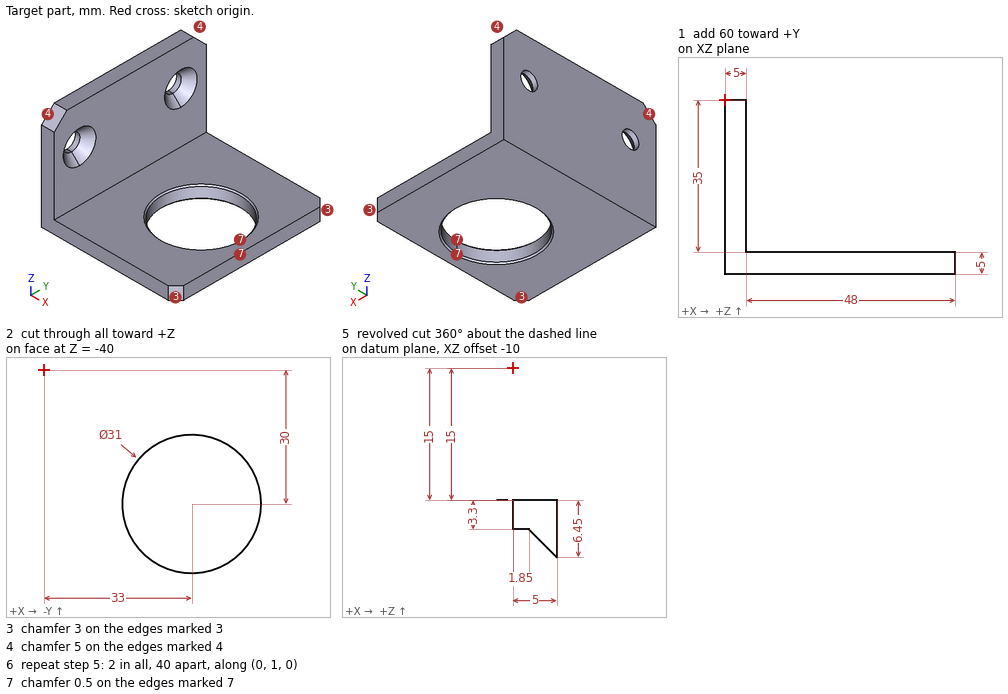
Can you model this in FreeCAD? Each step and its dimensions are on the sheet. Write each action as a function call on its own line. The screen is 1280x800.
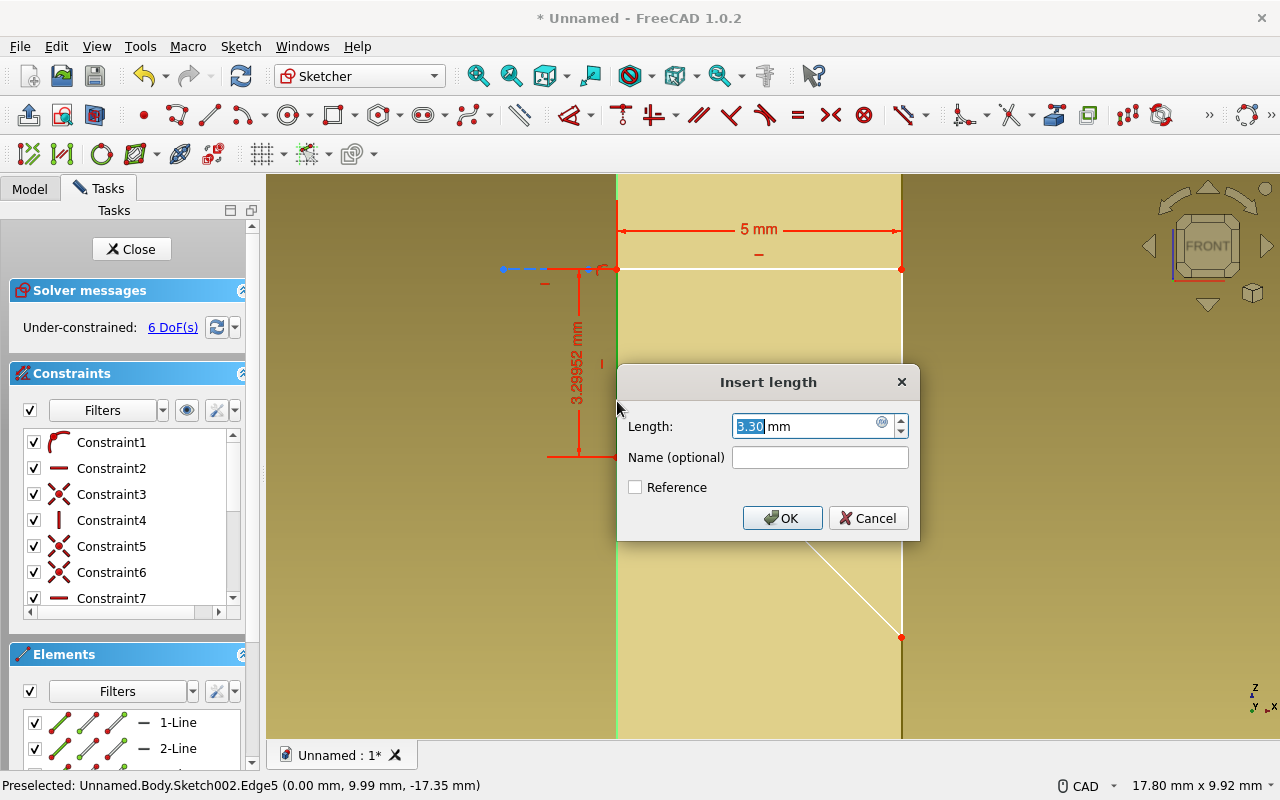
text(3.3)
key(Return)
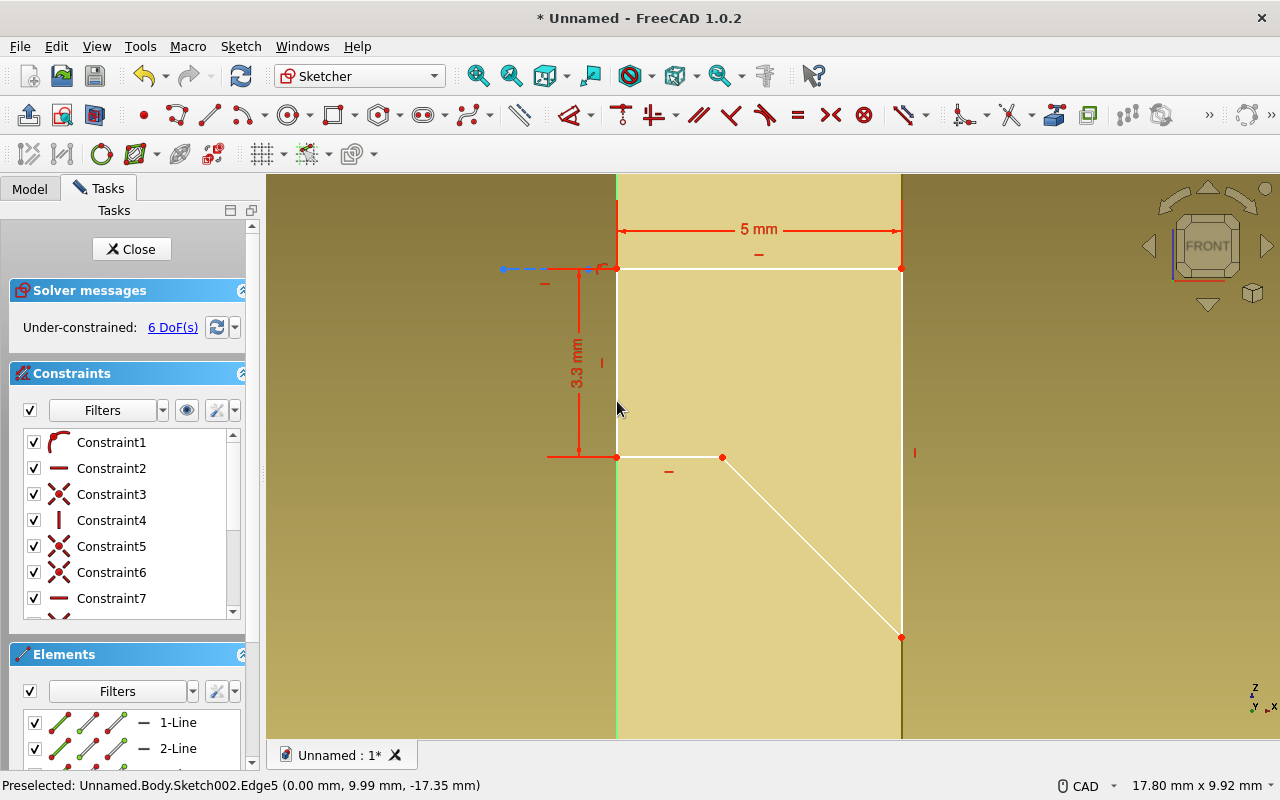
click(617, 269)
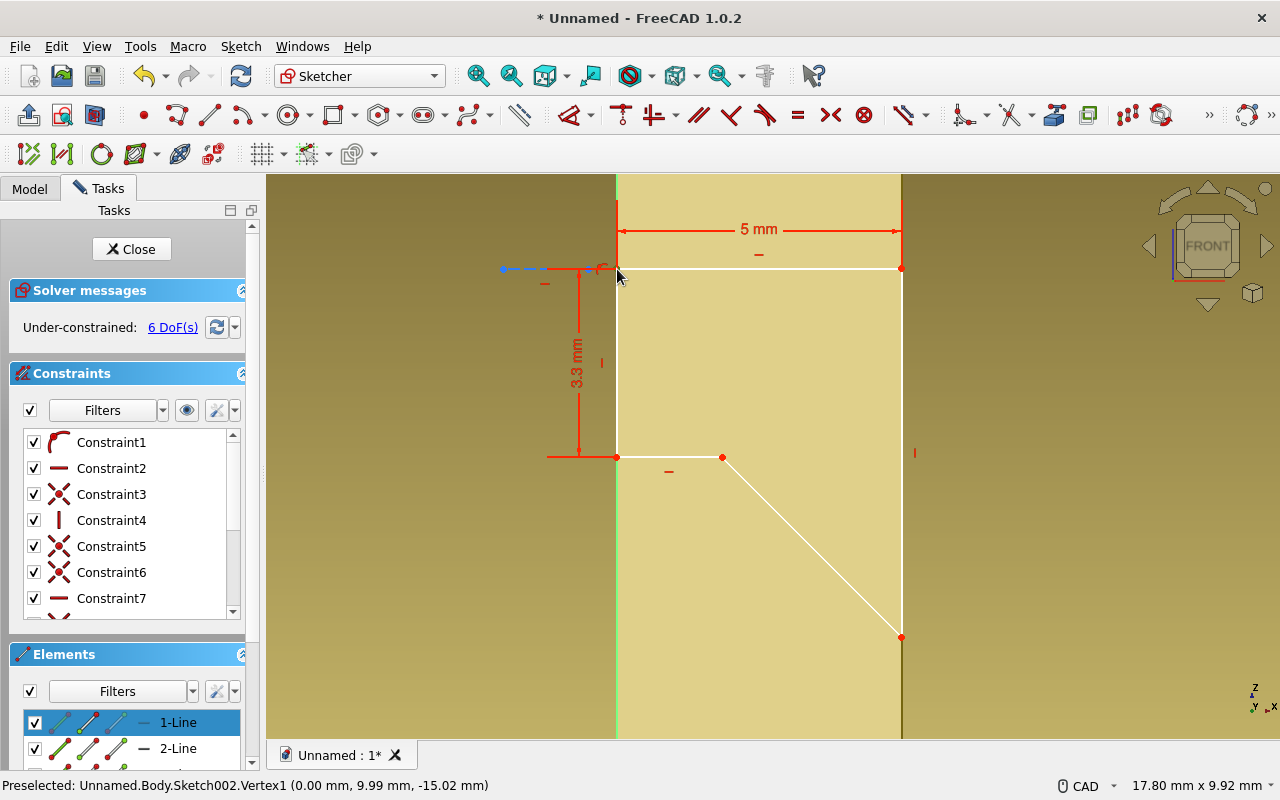
click(590, 116)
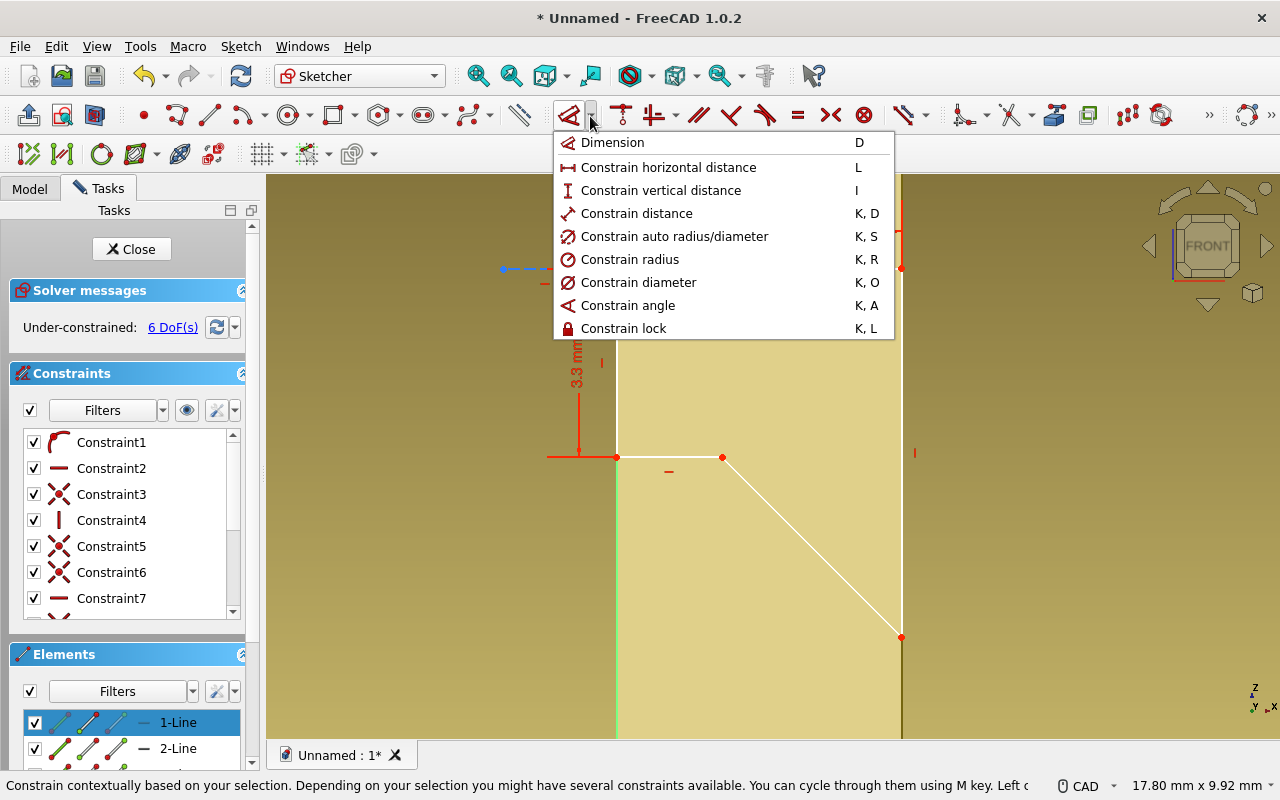
click(724, 190)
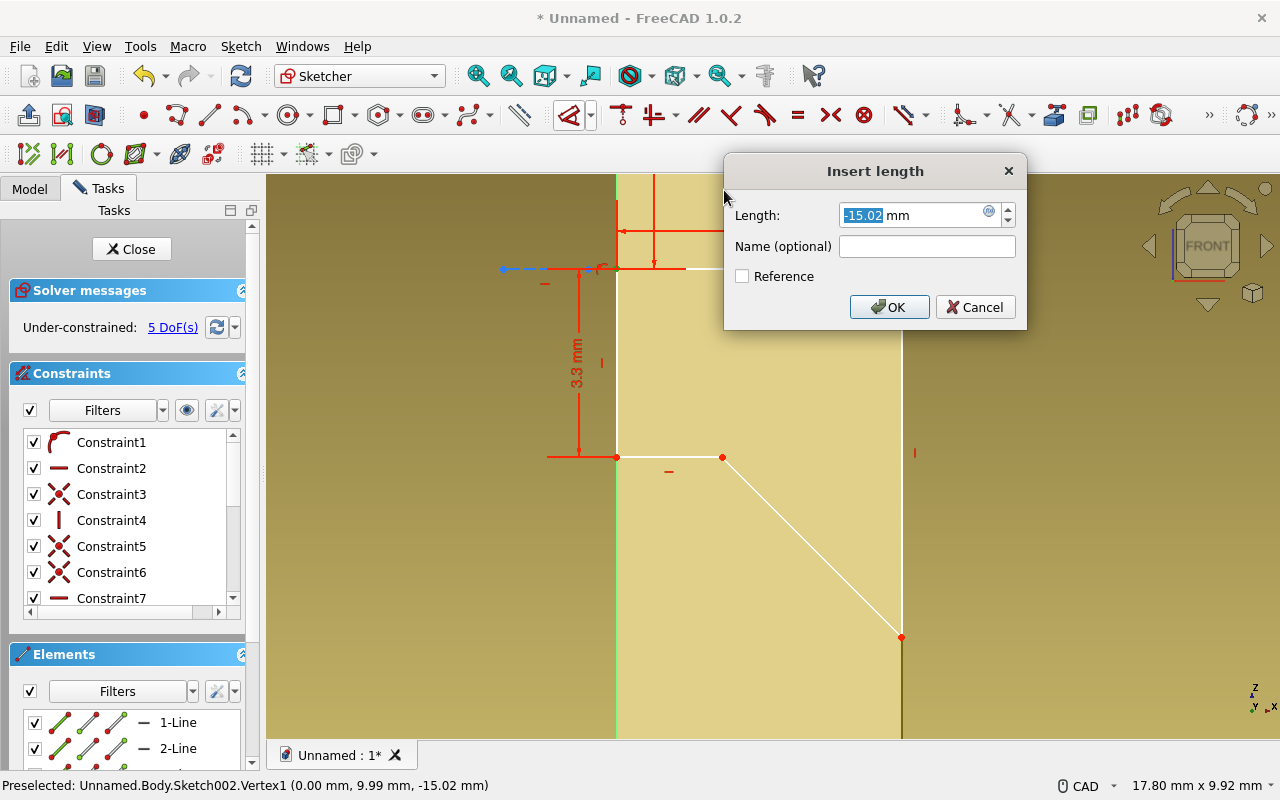
text(-15)
key(Return)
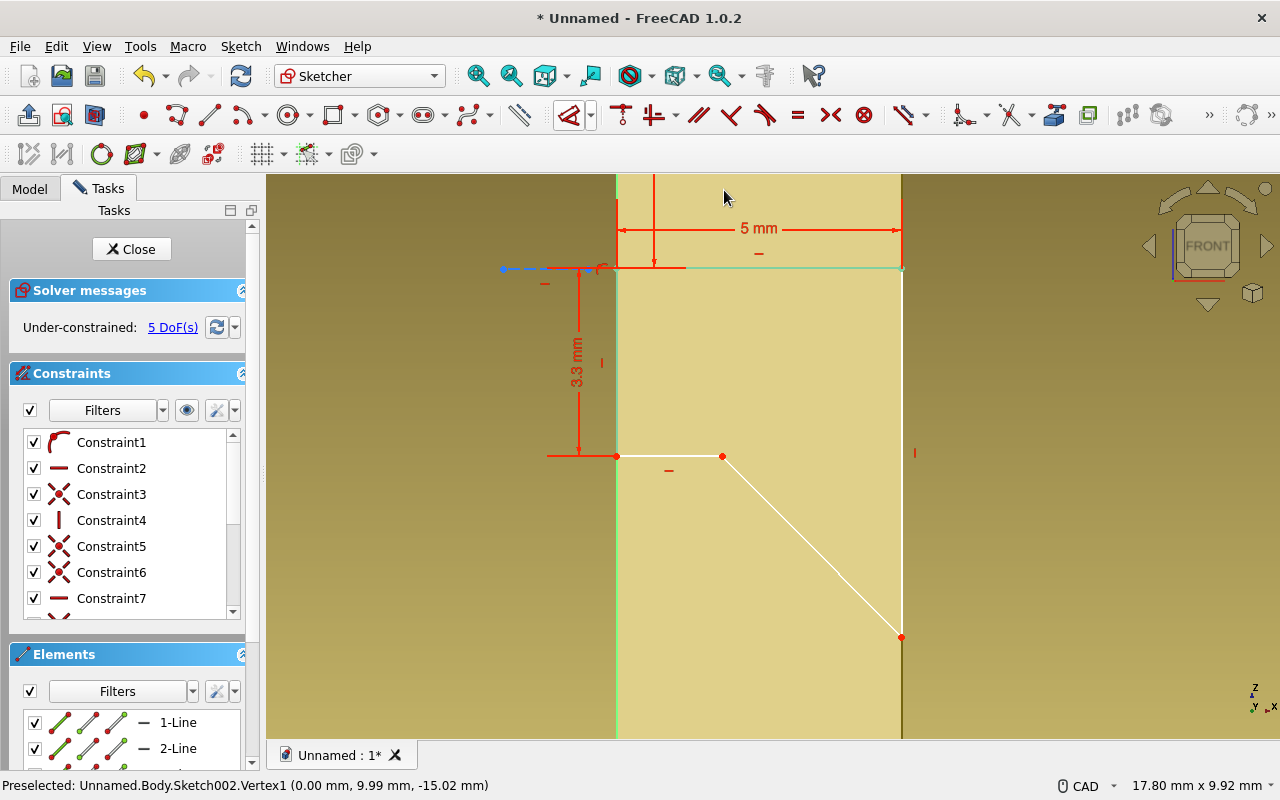
click(588, 269)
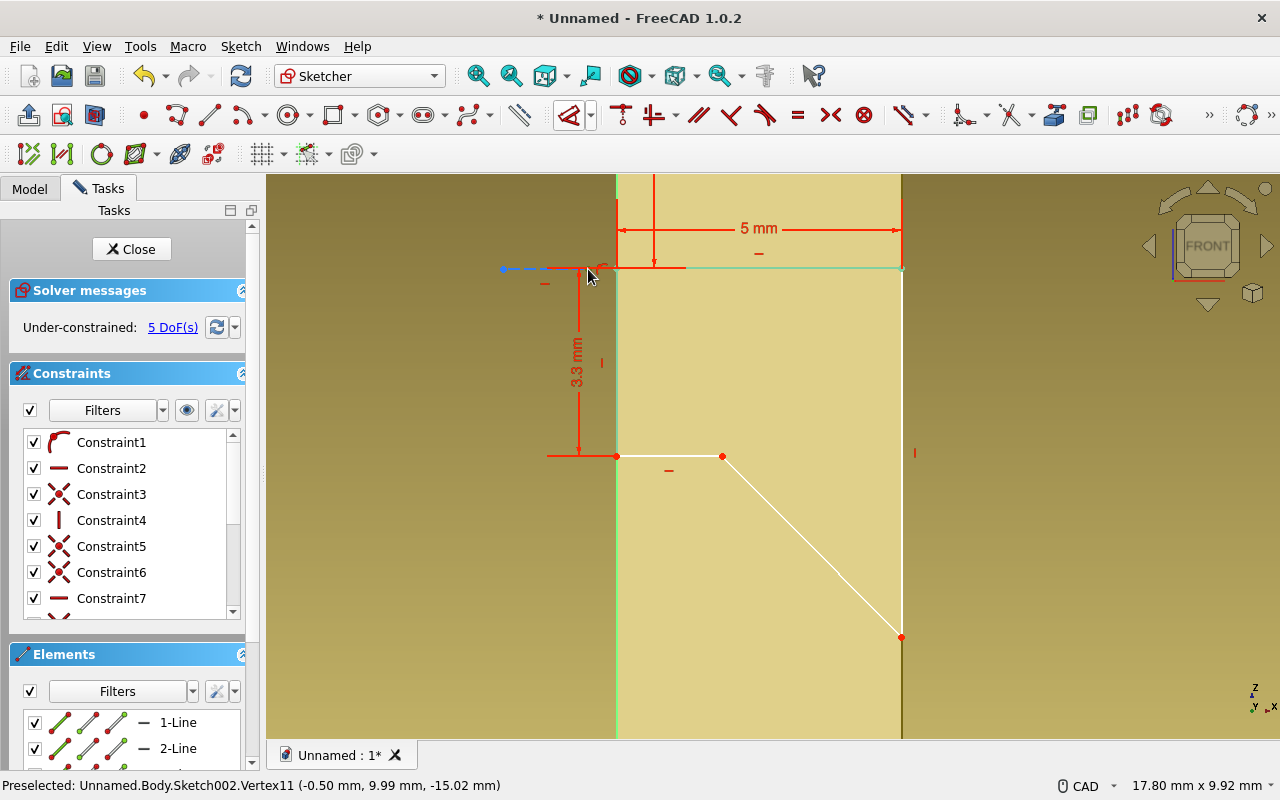
key(i)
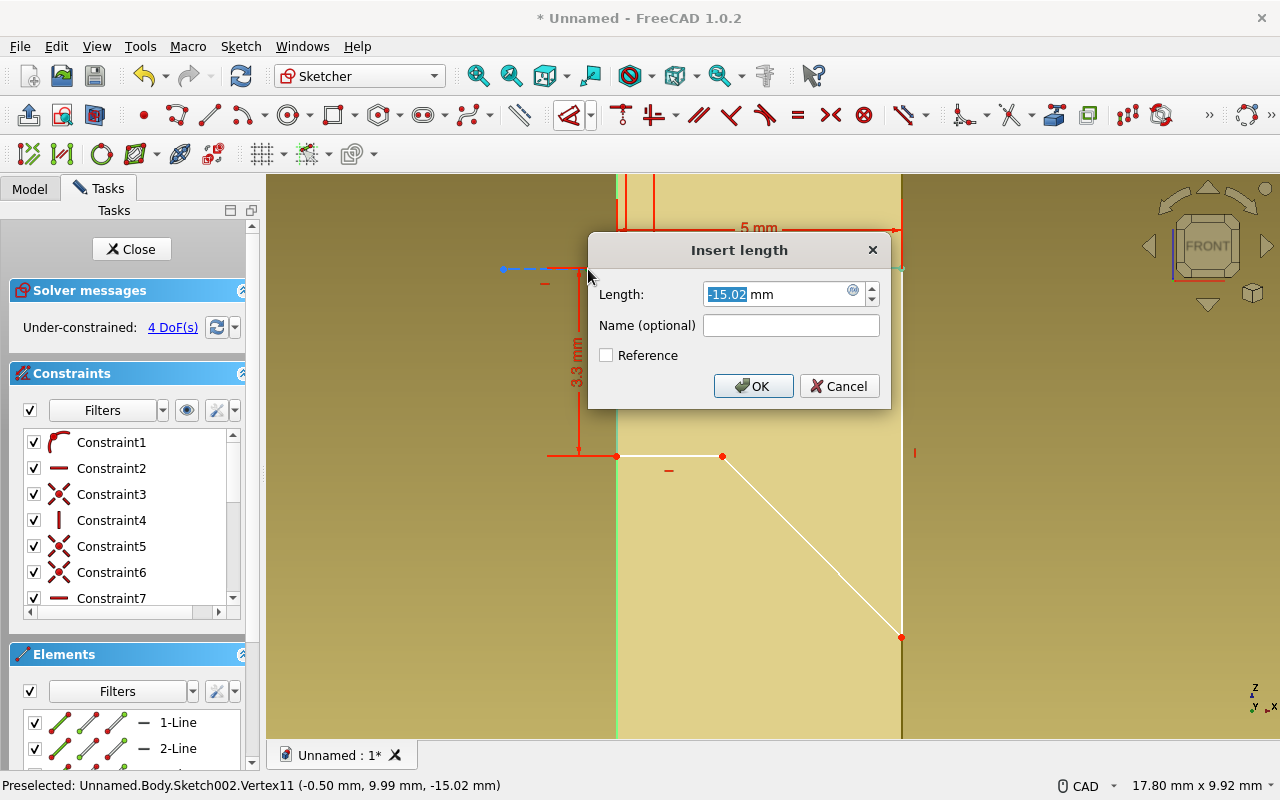
text(-15)
key(Return)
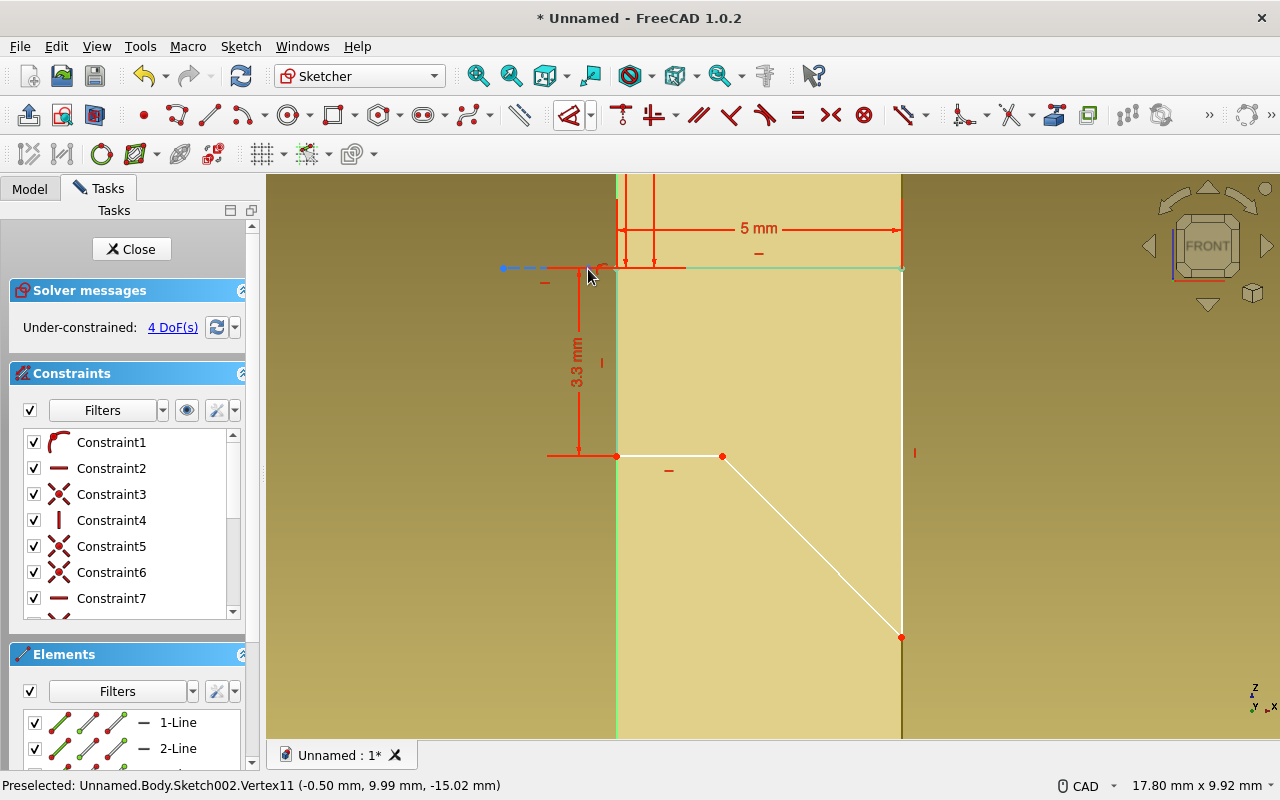
click(902, 379)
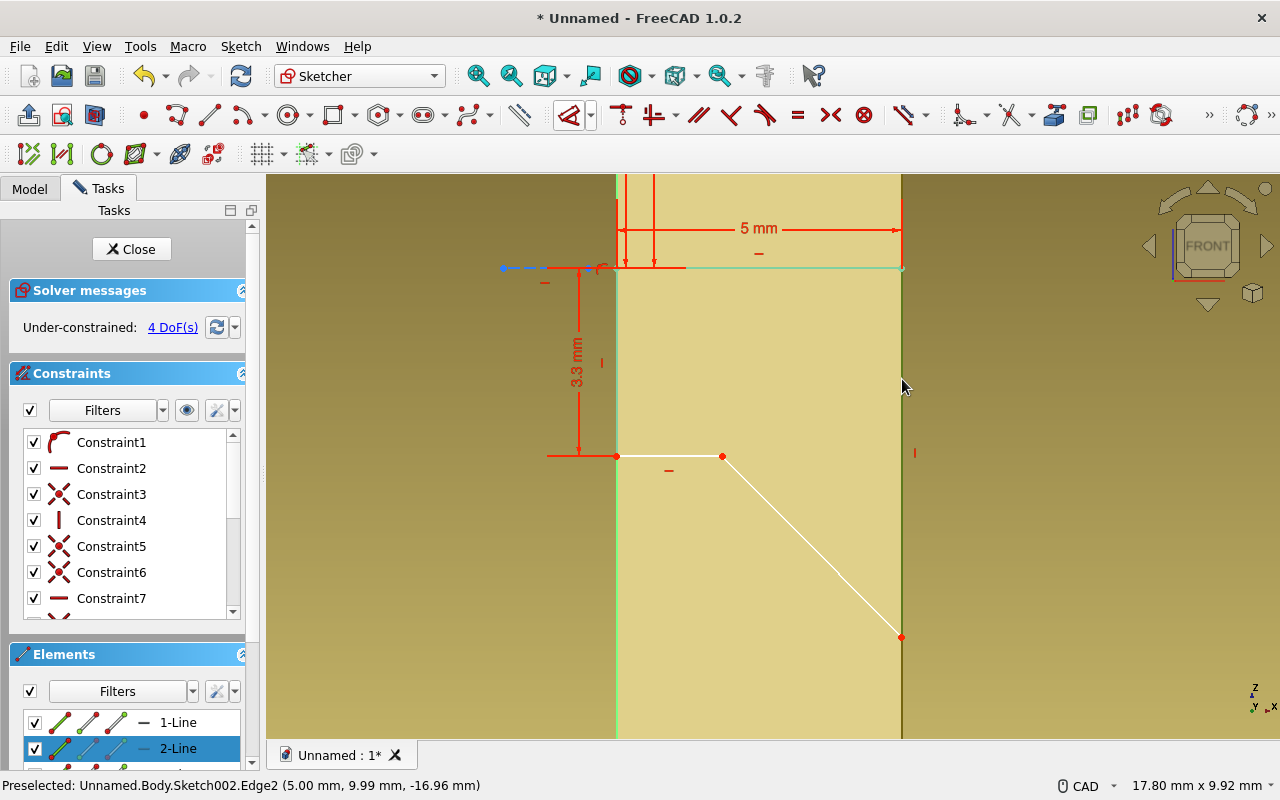
key(i)